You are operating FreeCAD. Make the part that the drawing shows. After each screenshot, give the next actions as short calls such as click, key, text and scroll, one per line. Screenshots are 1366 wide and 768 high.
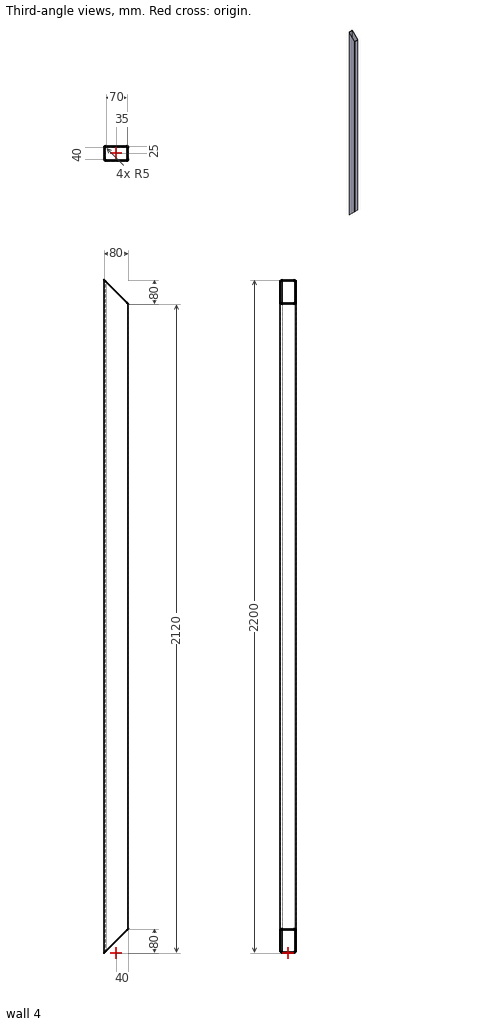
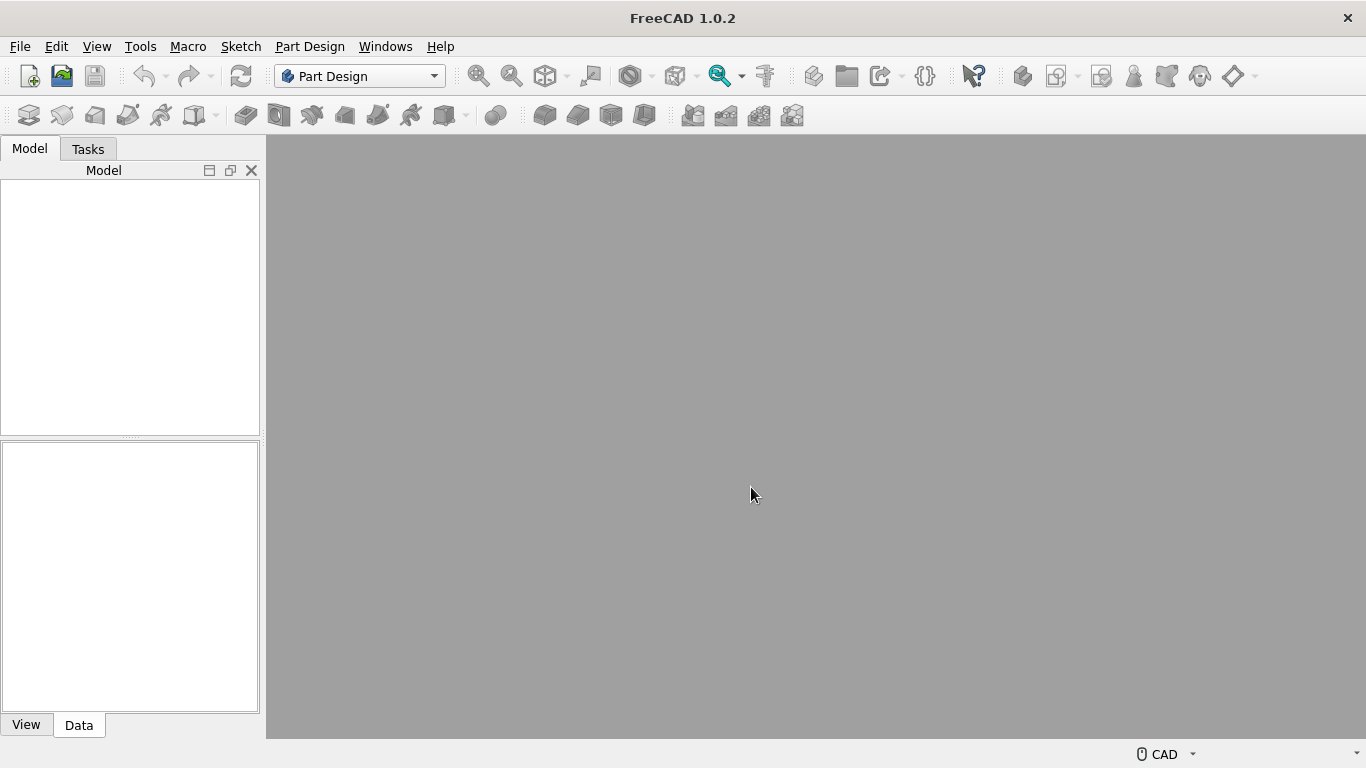
click(29, 76)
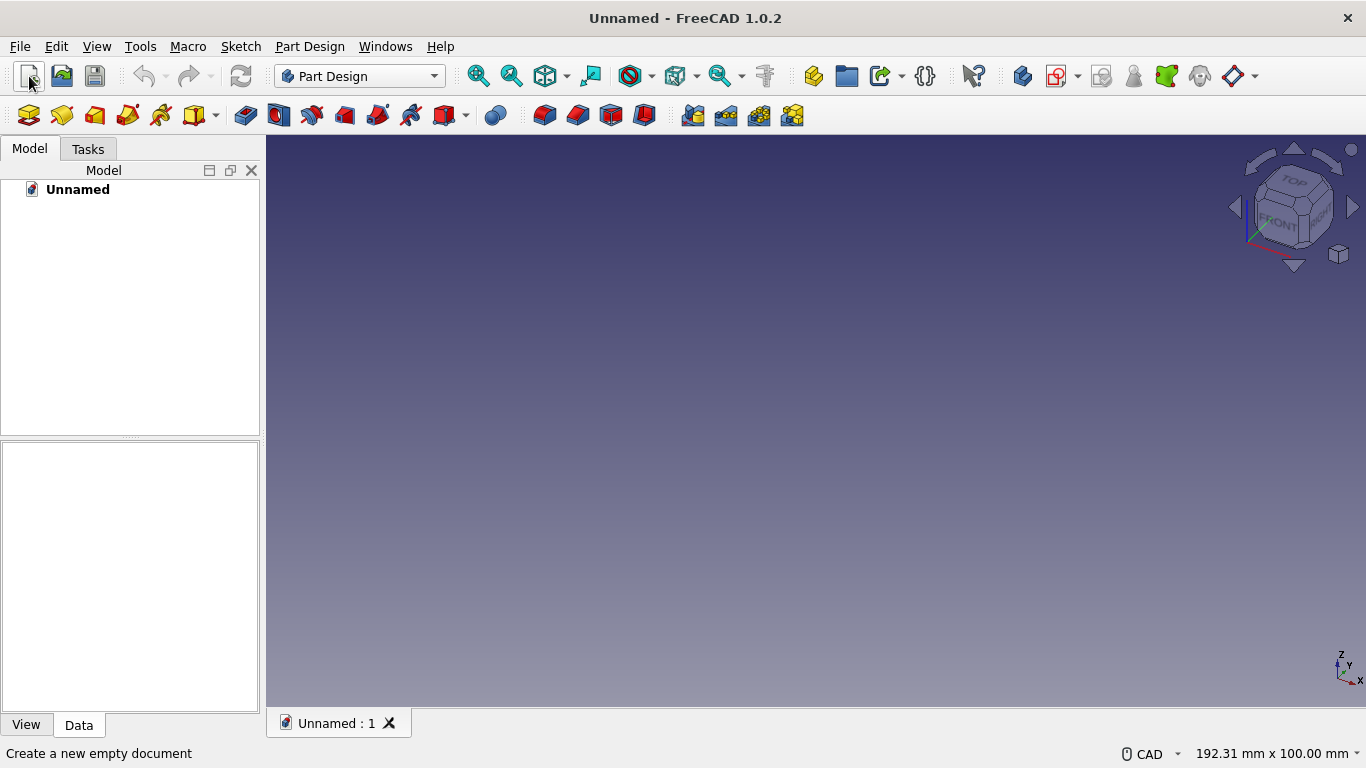
click(1056, 76)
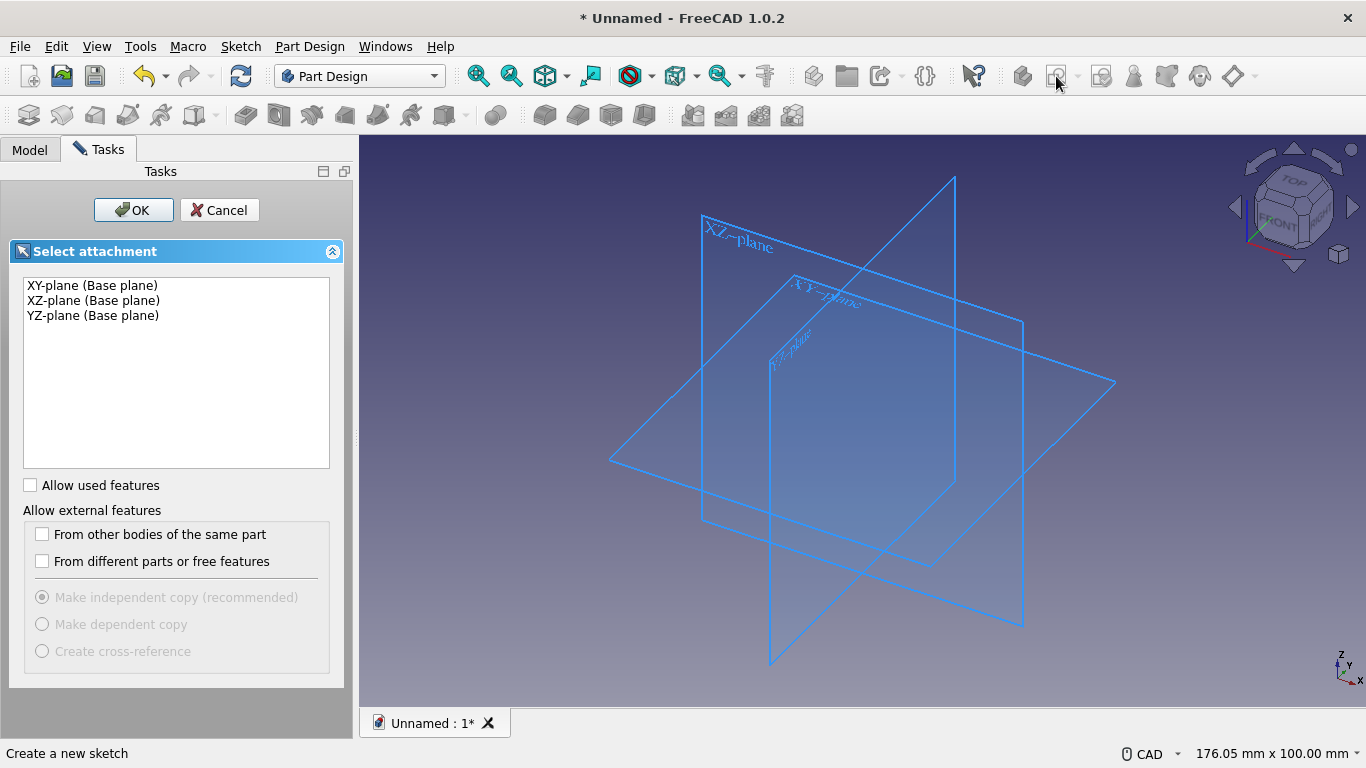
click(84, 286)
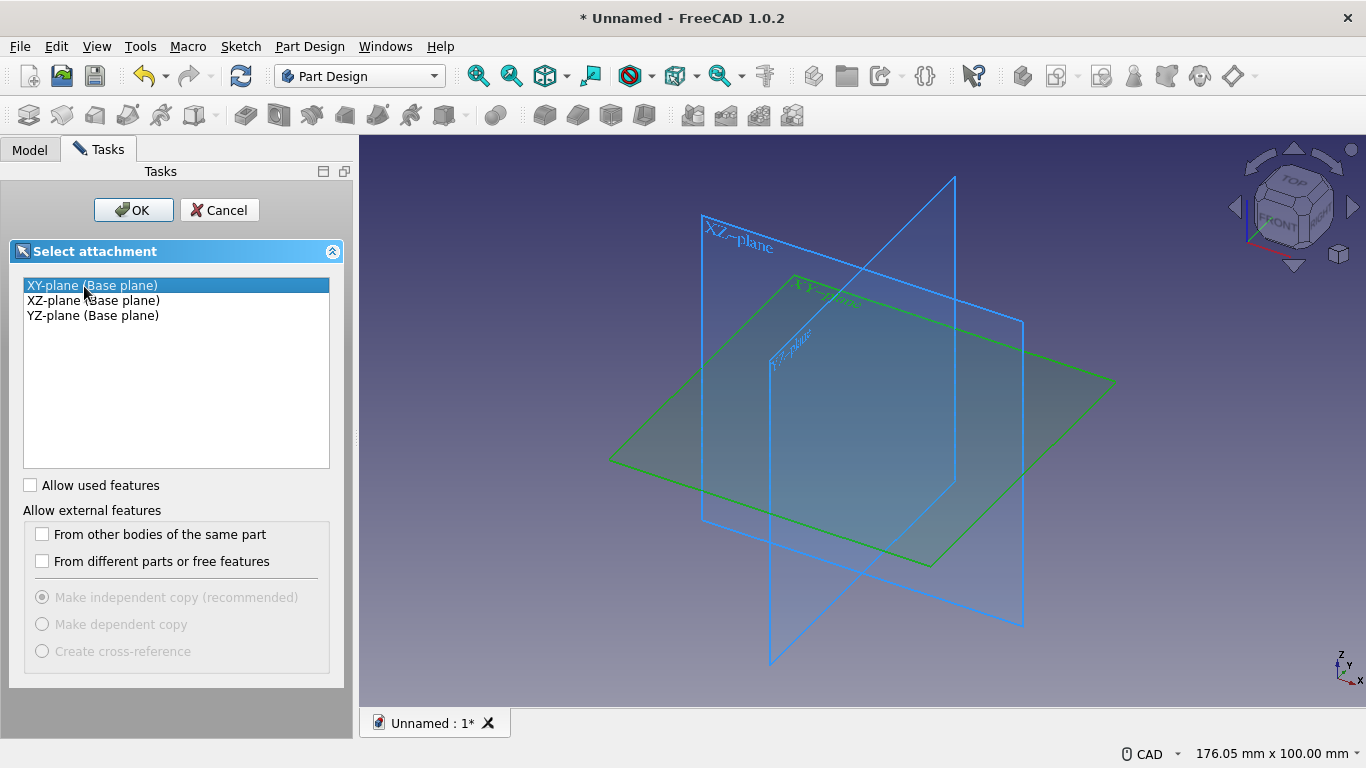
click(134, 210)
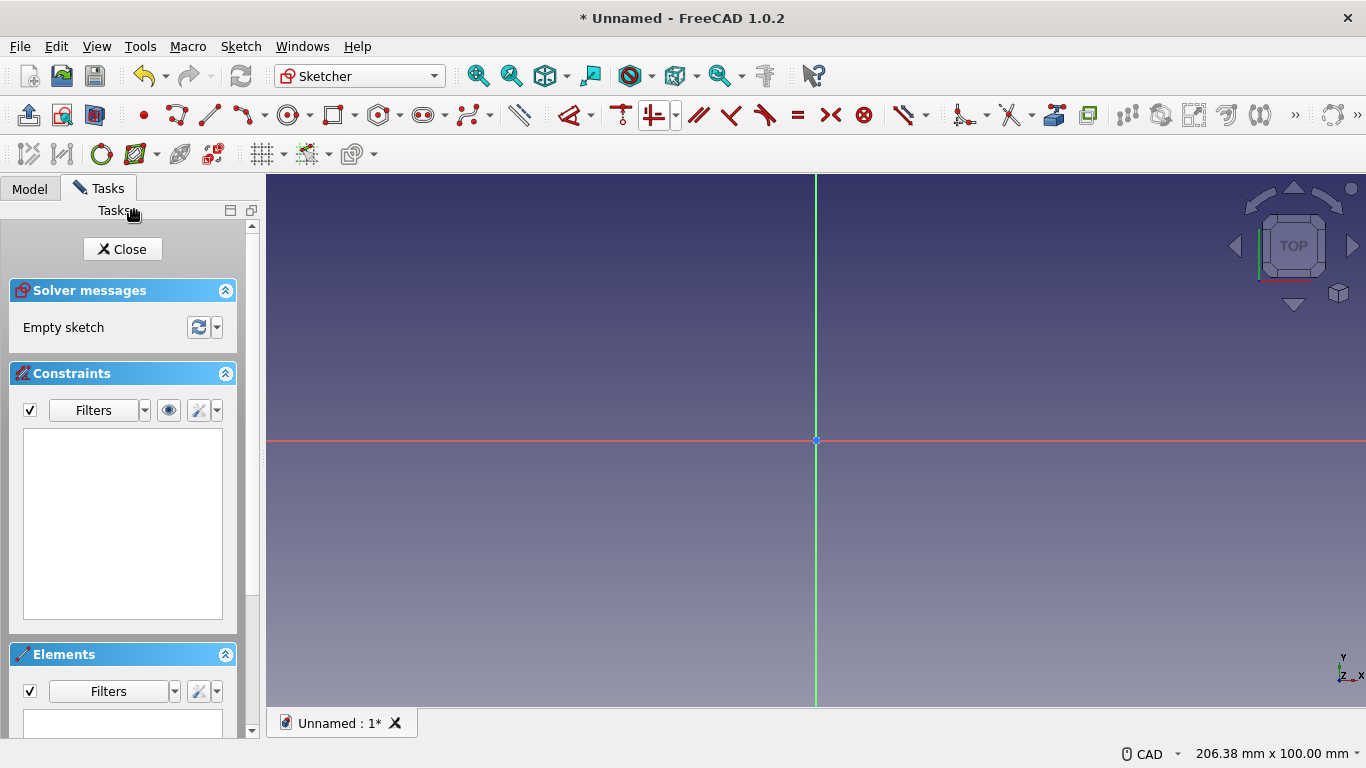
click(210, 116)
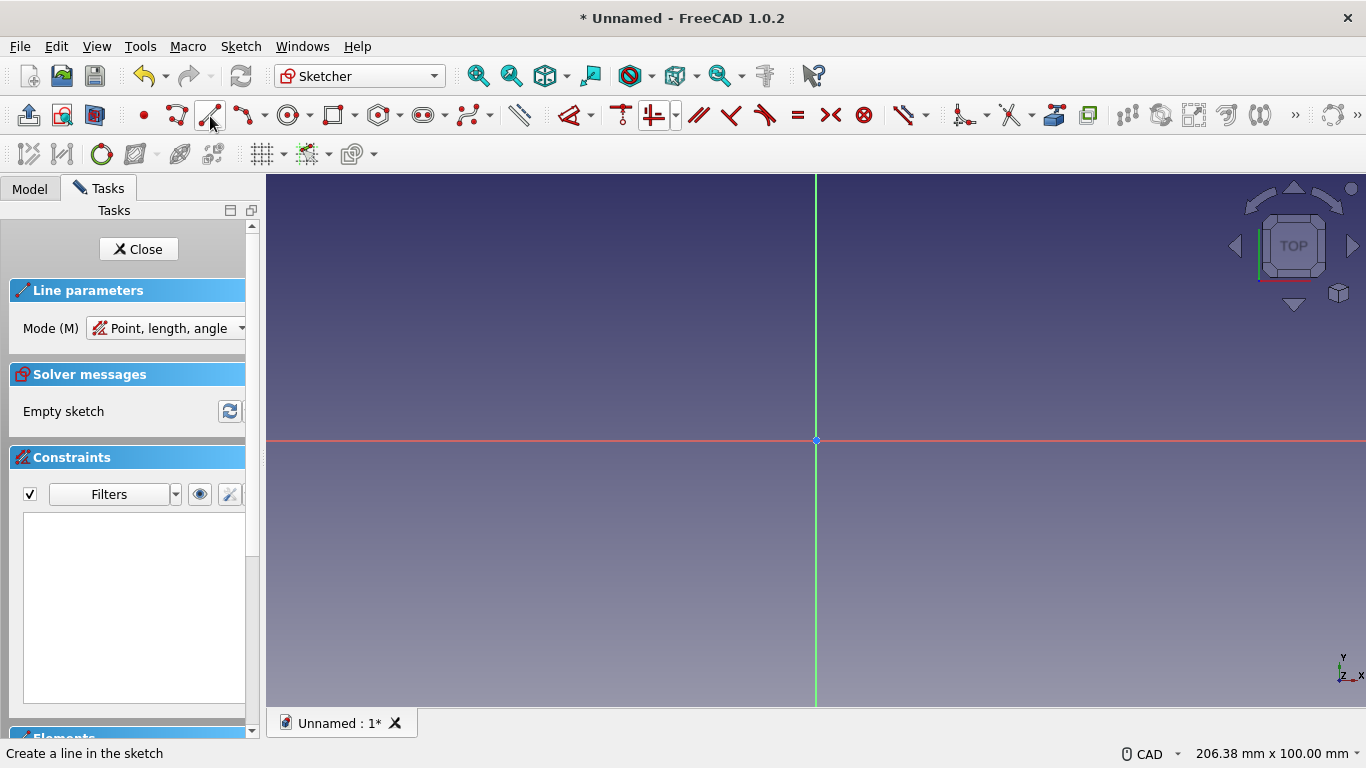
click(1003, 307)
click(629, 307)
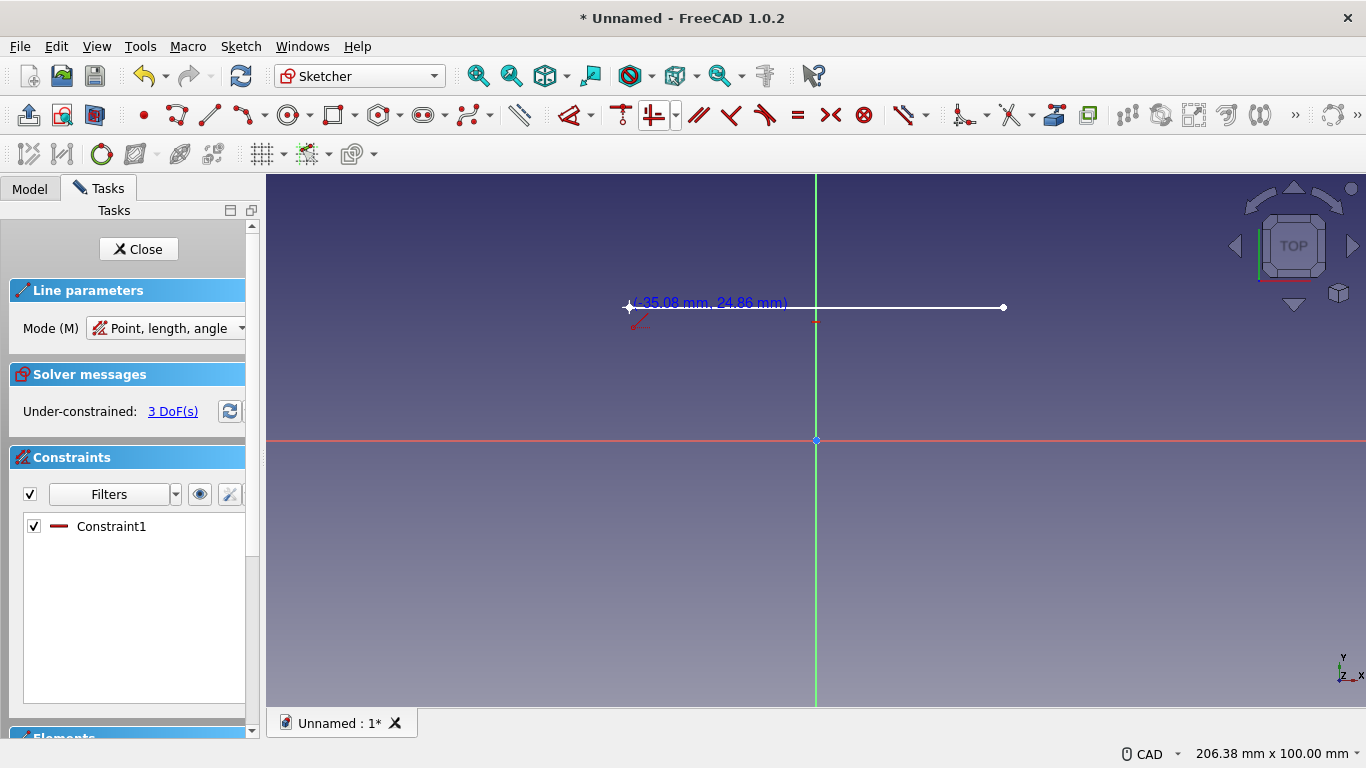
click(603, 334)
click(603, 547)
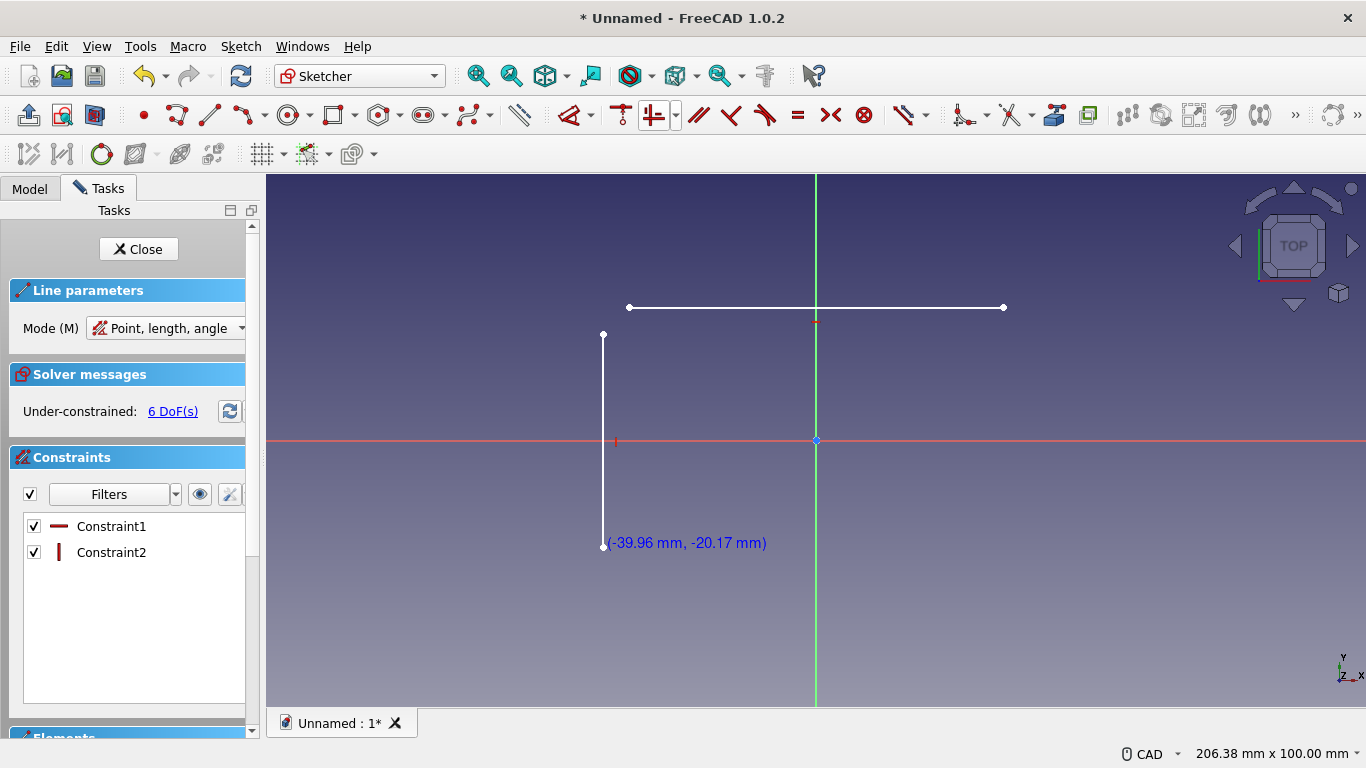
click(629, 574)
click(1003, 574)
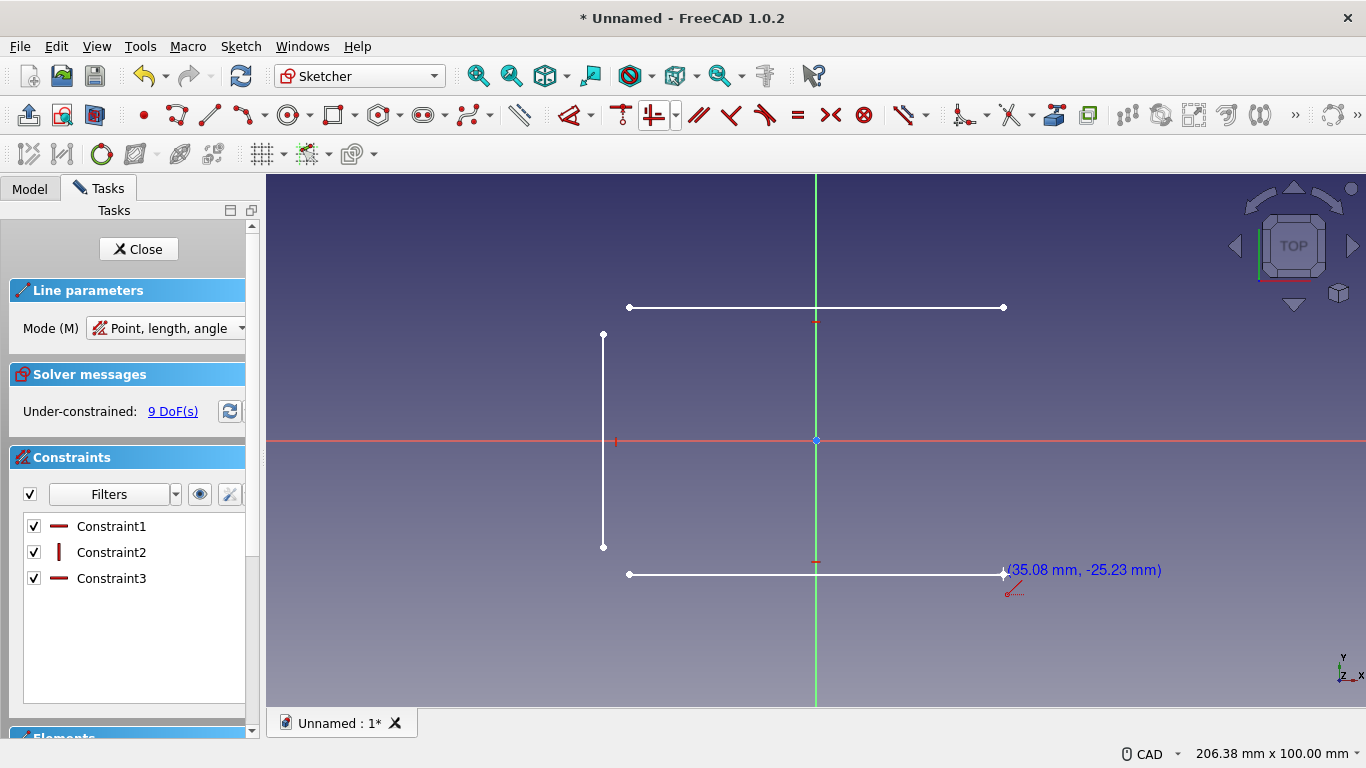
click(1029, 547)
click(1029, 334)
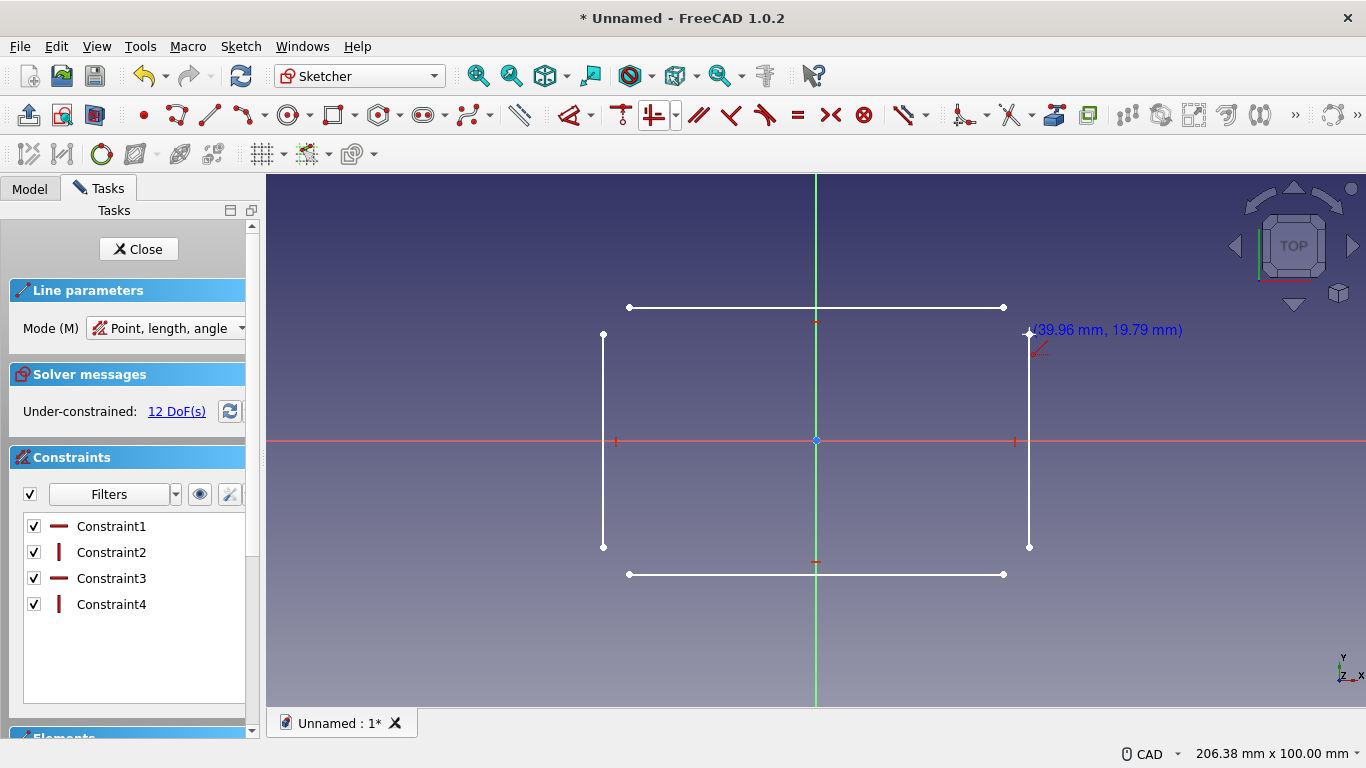
click(242, 116)